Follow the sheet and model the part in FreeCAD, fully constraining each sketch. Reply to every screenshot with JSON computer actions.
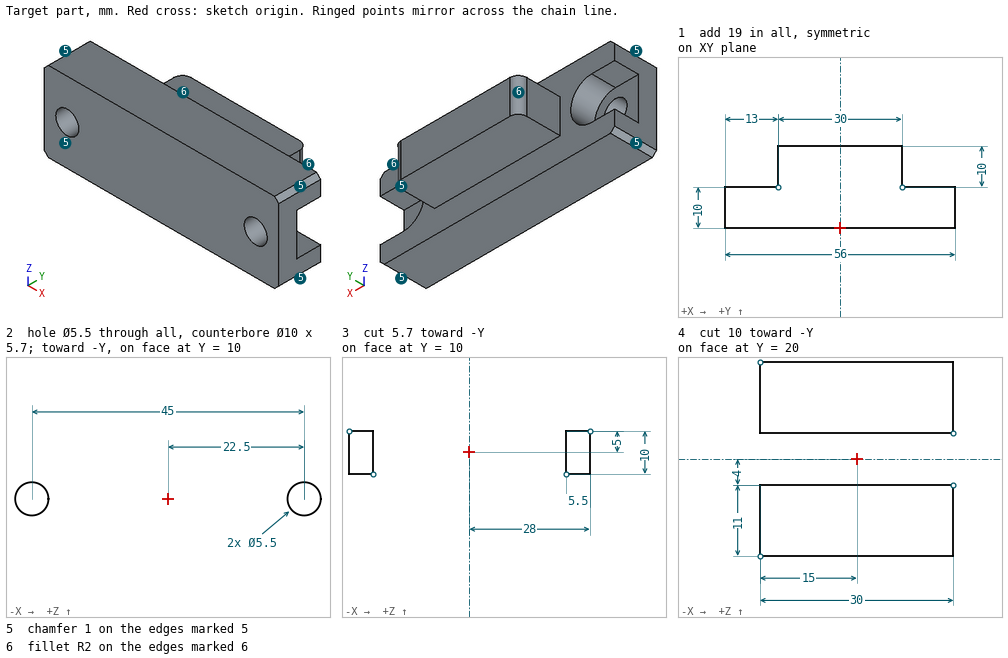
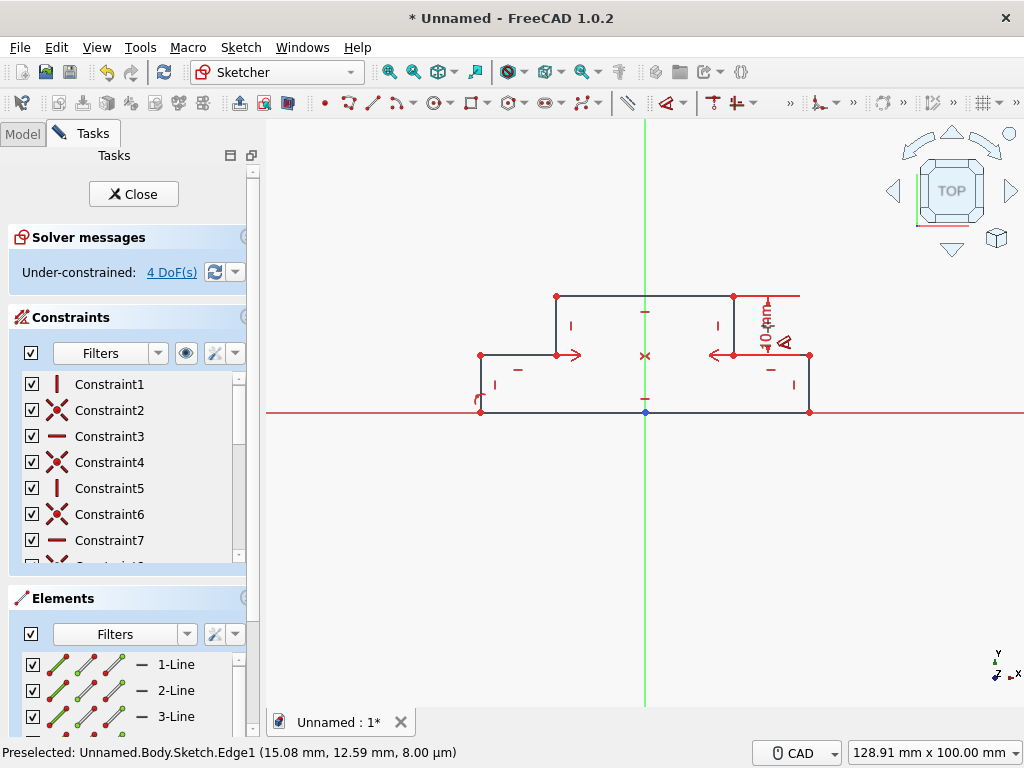
{"action": "left_click", "coordinate": [680, 296]}
{"action": "left_click", "coordinate": [604, 262]}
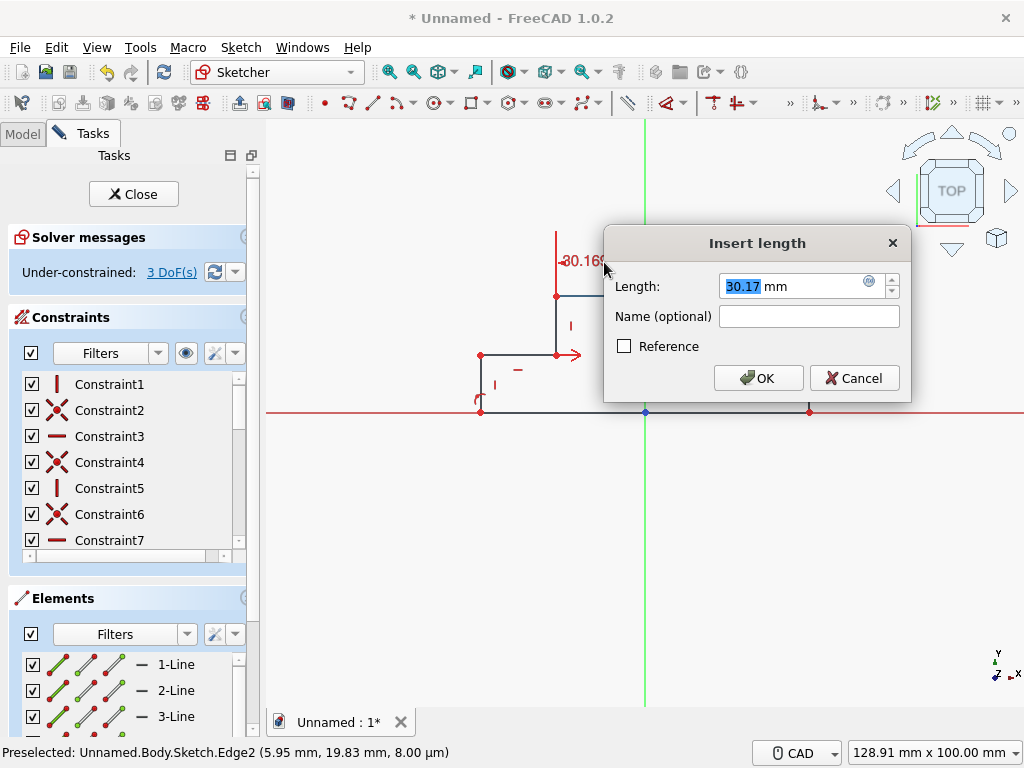
{"action": "type", "text": "30"}
{"action": "key", "text": "Return"}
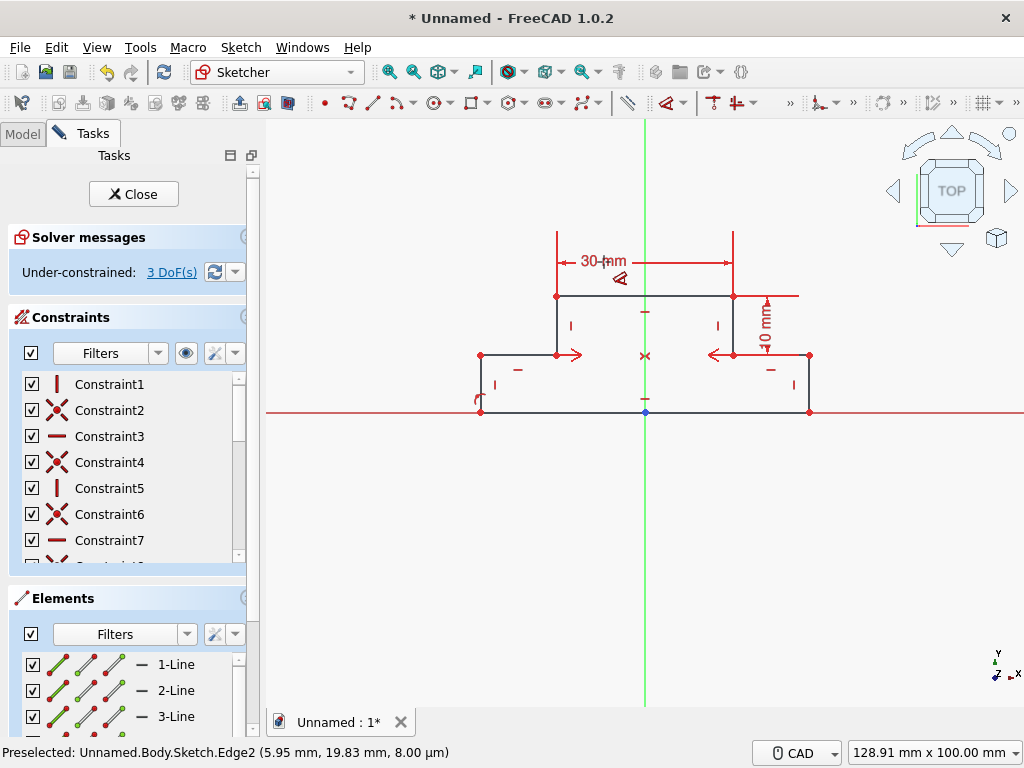
{"action": "left_click", "coordinate": [534, 355]}
{"action": "left_click", "coordinate": [519, 389]}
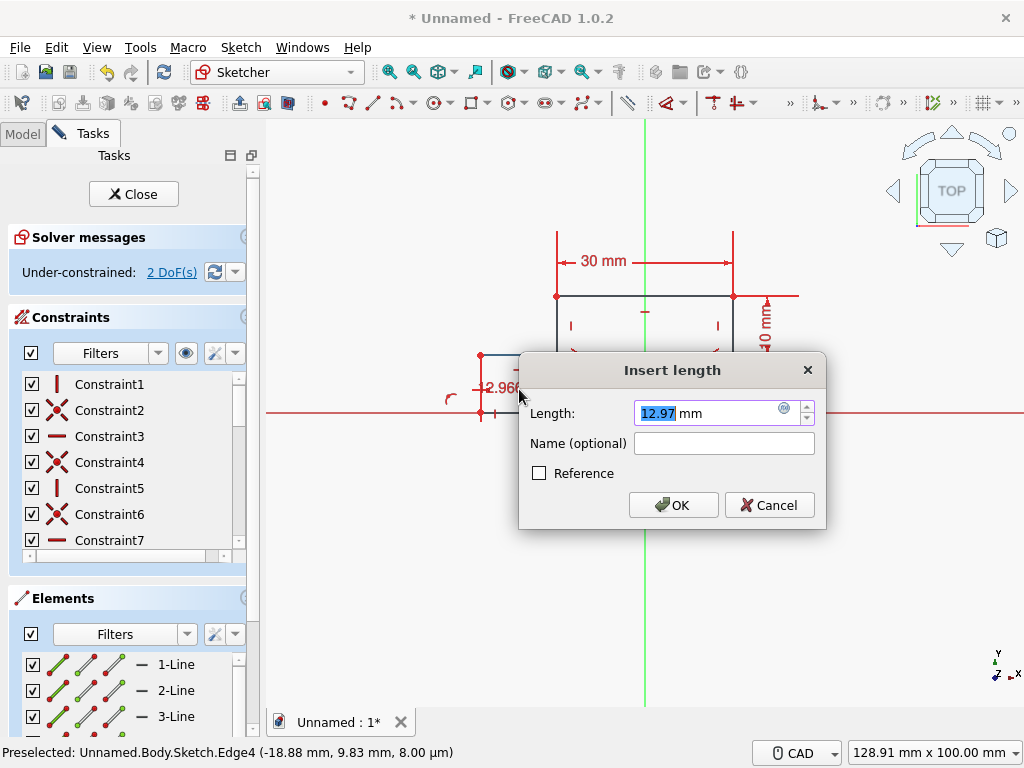
{"action": "type", "text": "13"}
{"action": "key", "text": "Return"}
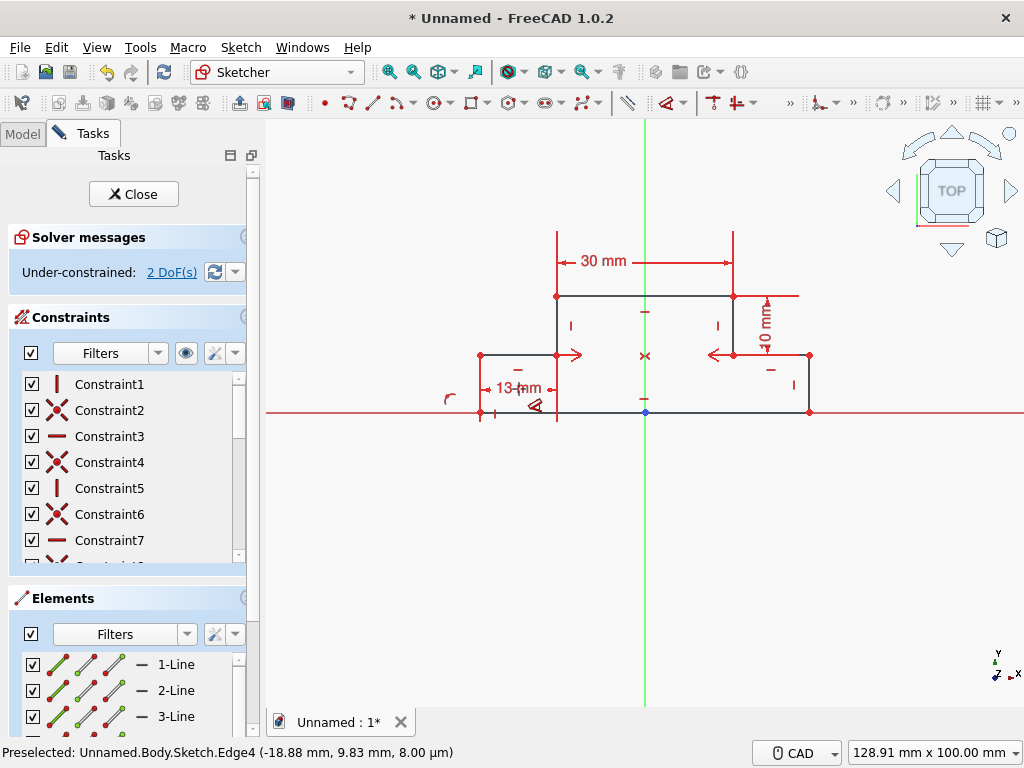
{"action": "left_click", "coordinate": [480, 373]}
{"action": "left_click", "coordinate": [446, 384]}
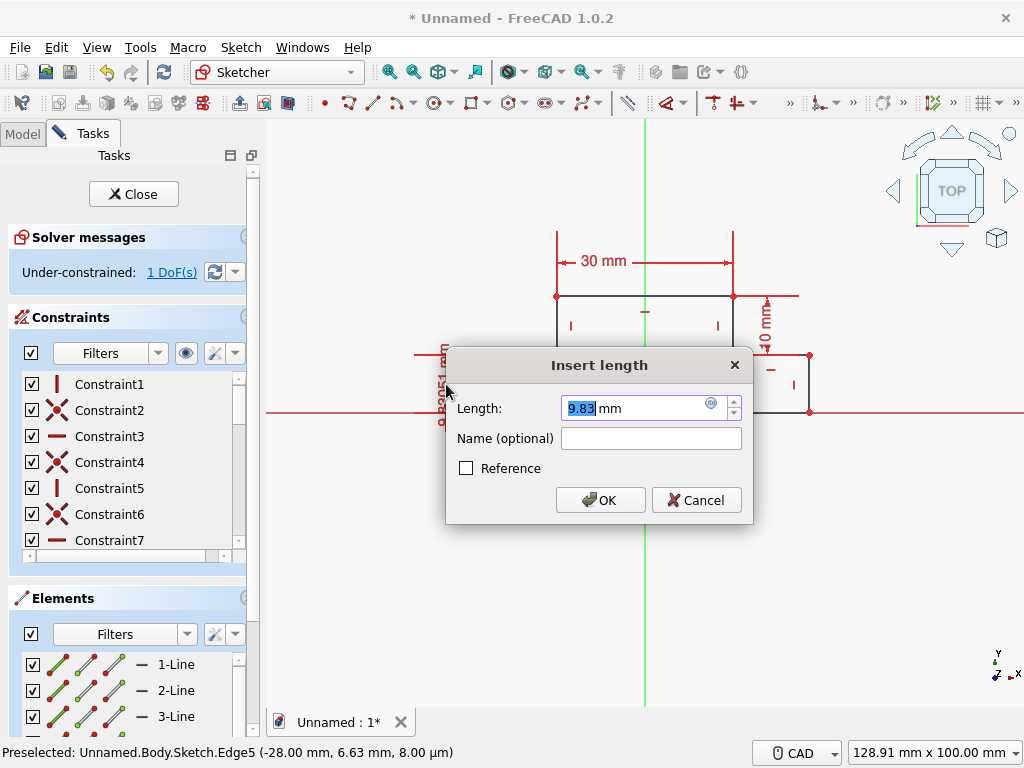
{"action": "type", "text": "10"}
{"action": "key", "text": "Return"}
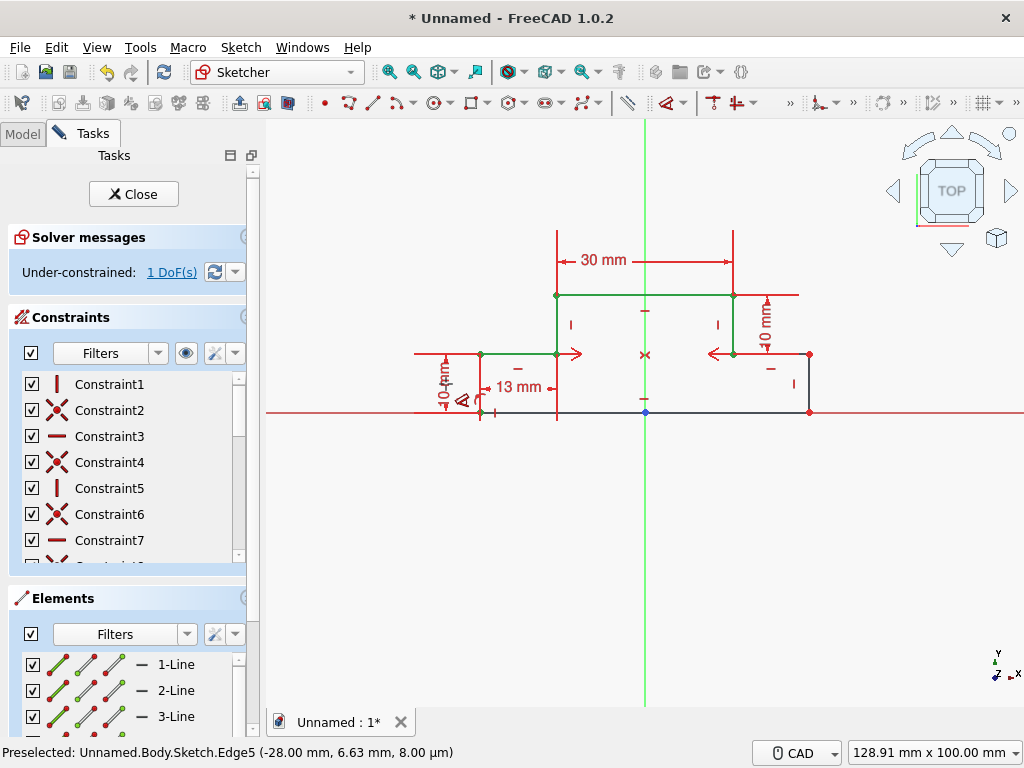
{"action": "left_click", "coordinate": [579, 413]}
{"action": "left_click", "coordinate": [569, 447]}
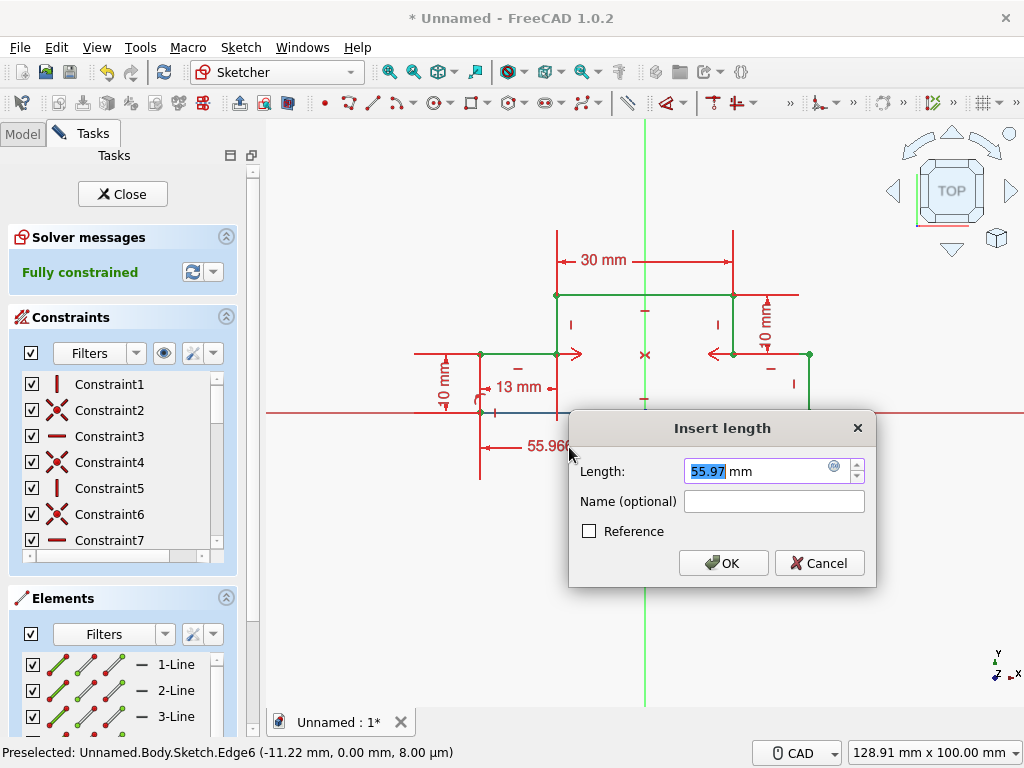
{"action": "type", "text": "56"}
{"action": "key", "text": "Return"}
{"action": "key", "text": "Escape"}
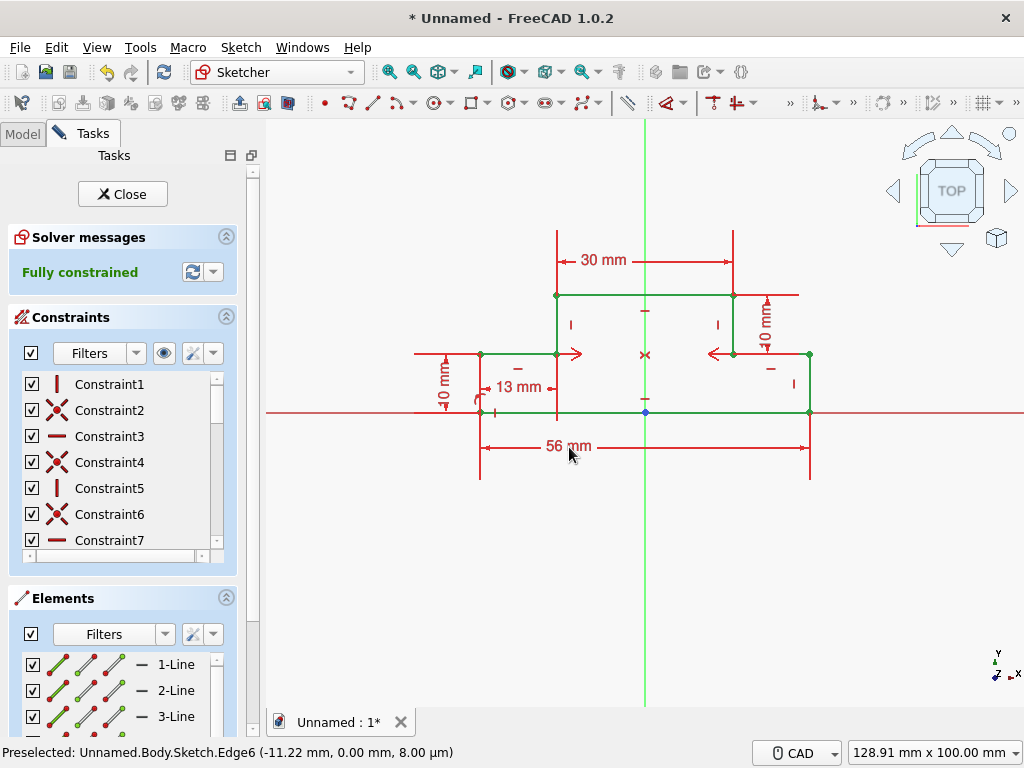
{"action": "left_click", "coordinate": [123, 194]}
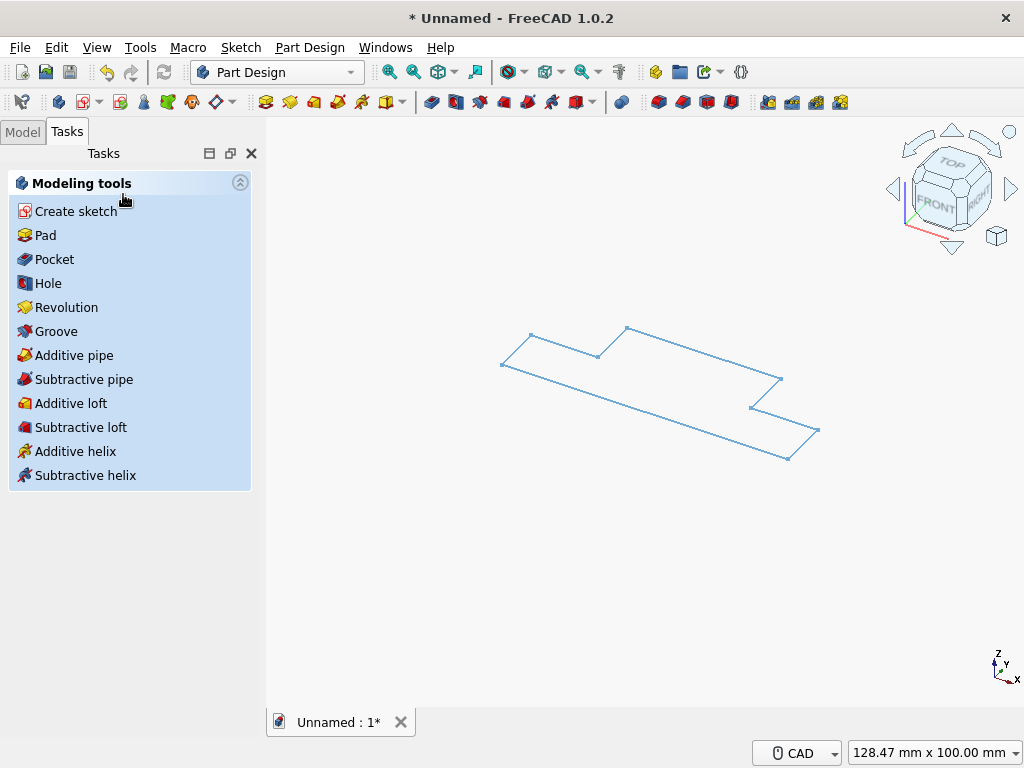
{"action": "left_click", "coordinate": [266, 102]}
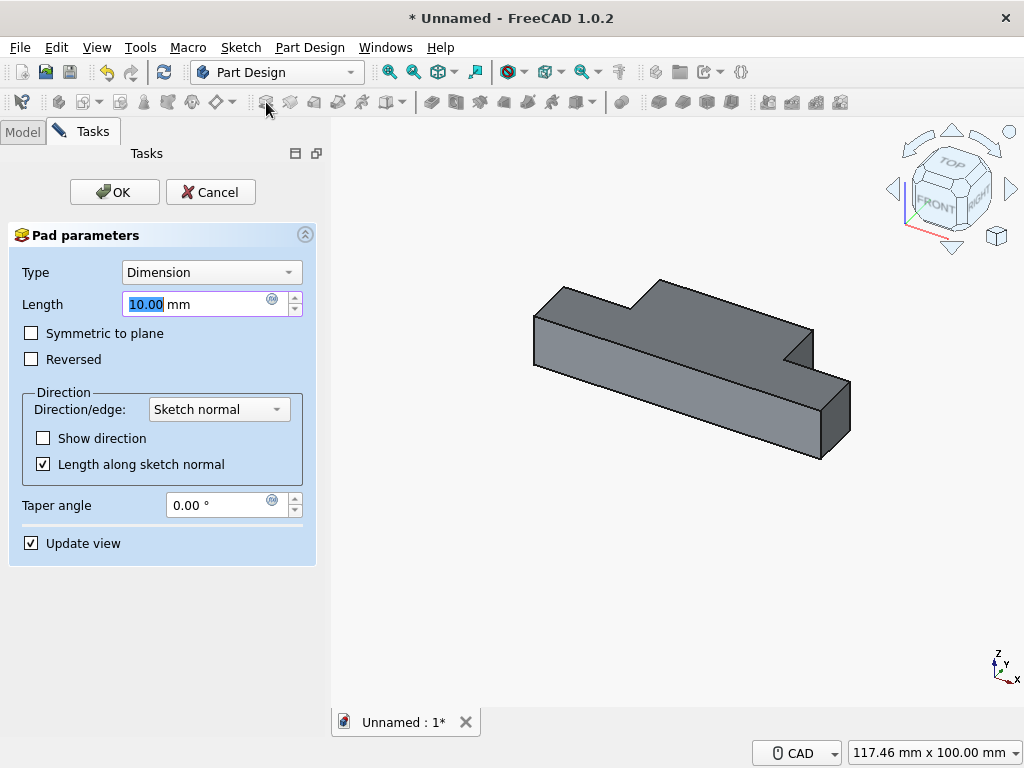
{"action": "type", "text": "19"}
{"action": "key", "text": "Tab"}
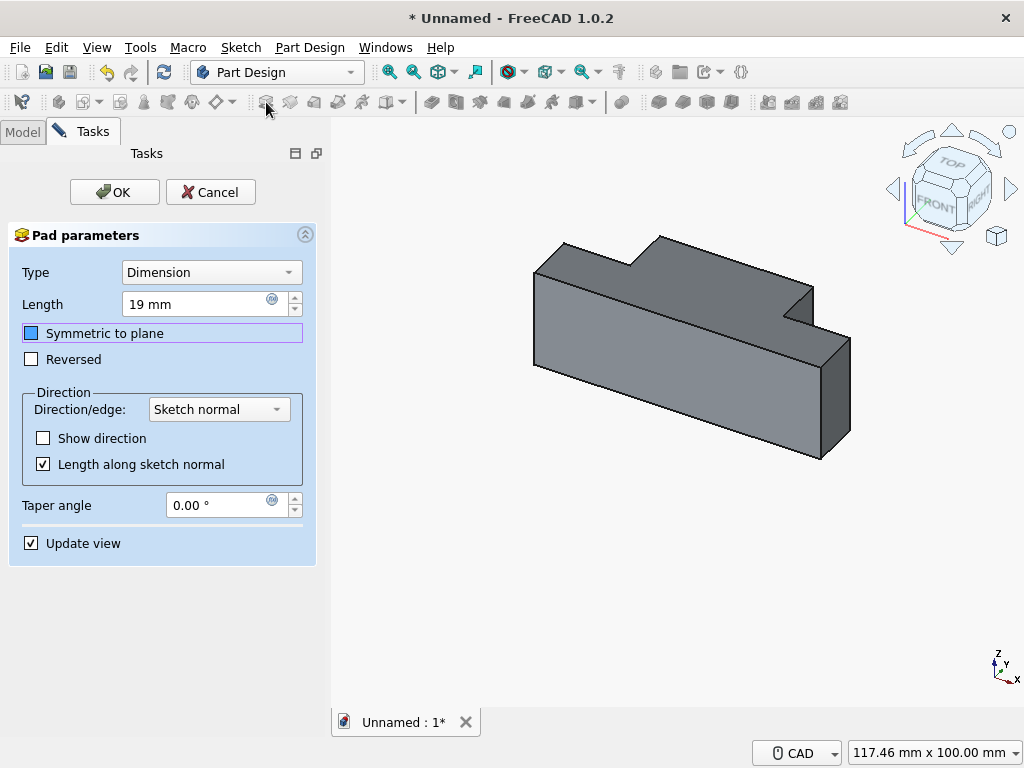
{"action": "left_click", "coordinate": [30, 333]}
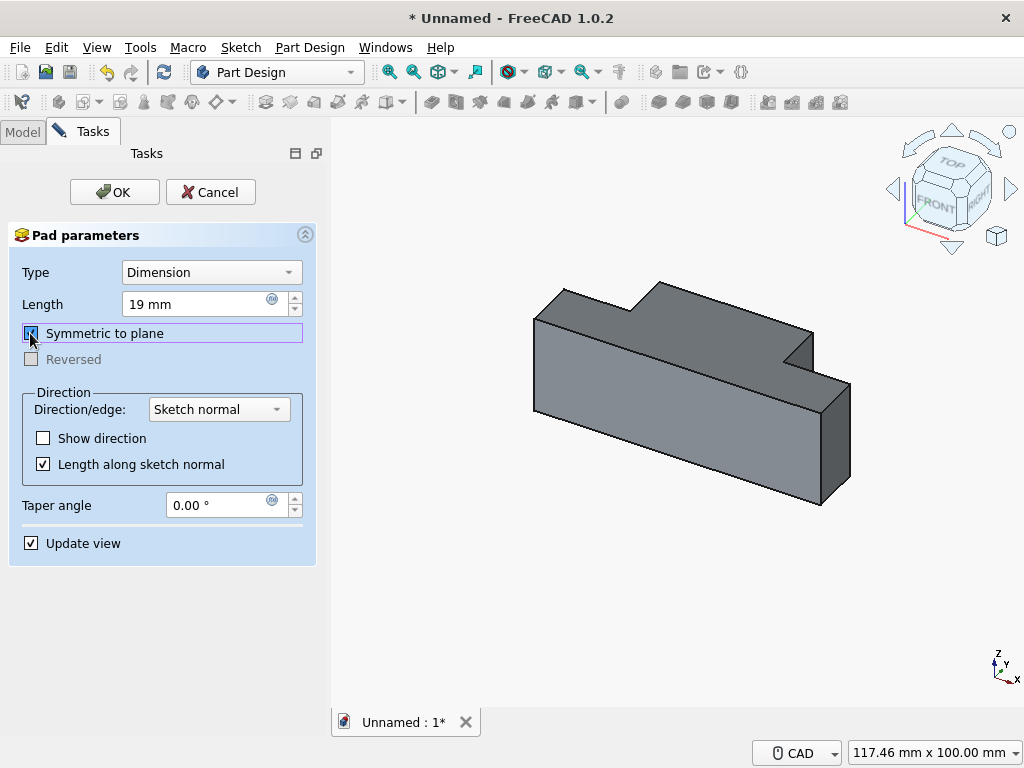
{"action": "left_click", "coordinate": [115, 192]}